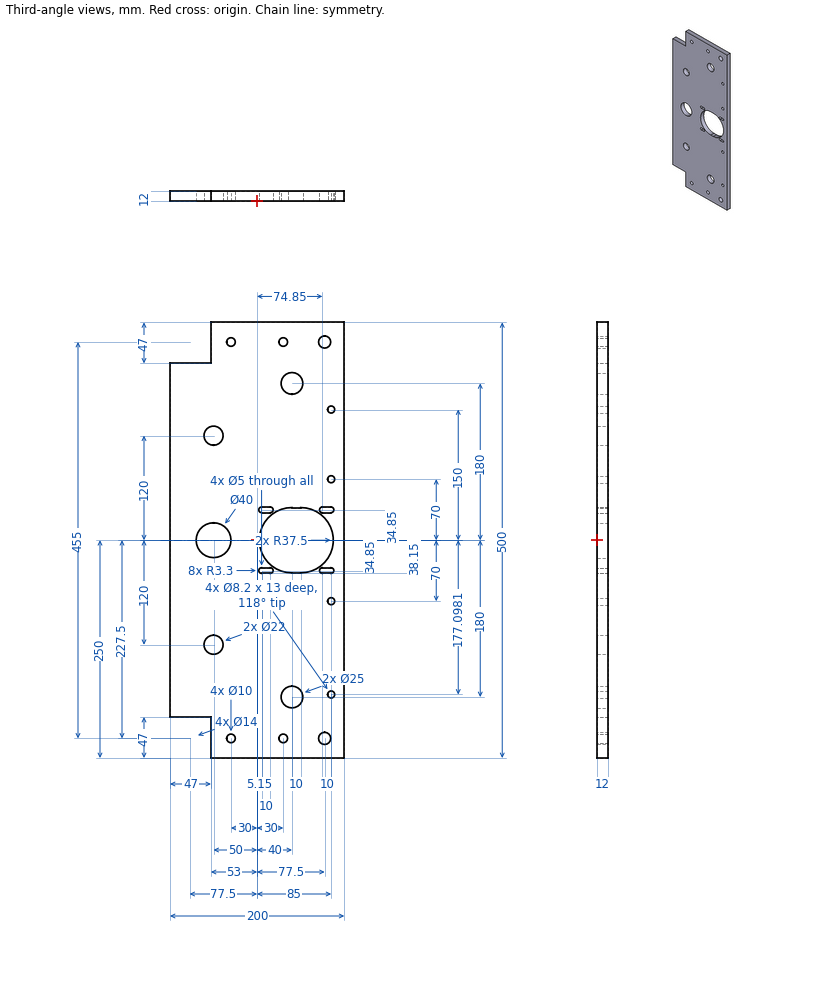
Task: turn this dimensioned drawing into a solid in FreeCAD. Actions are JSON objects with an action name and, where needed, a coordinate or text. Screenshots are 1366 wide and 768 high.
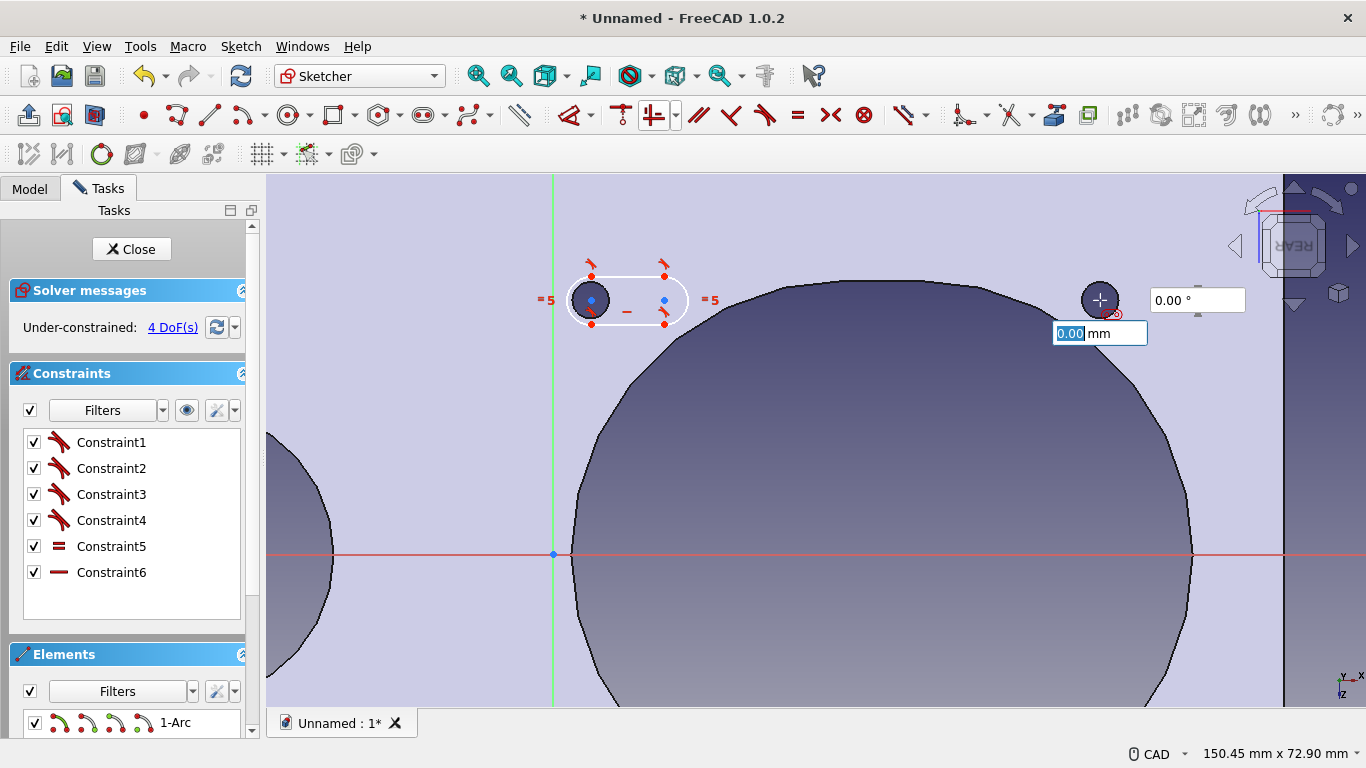
{"action": "left_click", "coordinate": [1173, 300]}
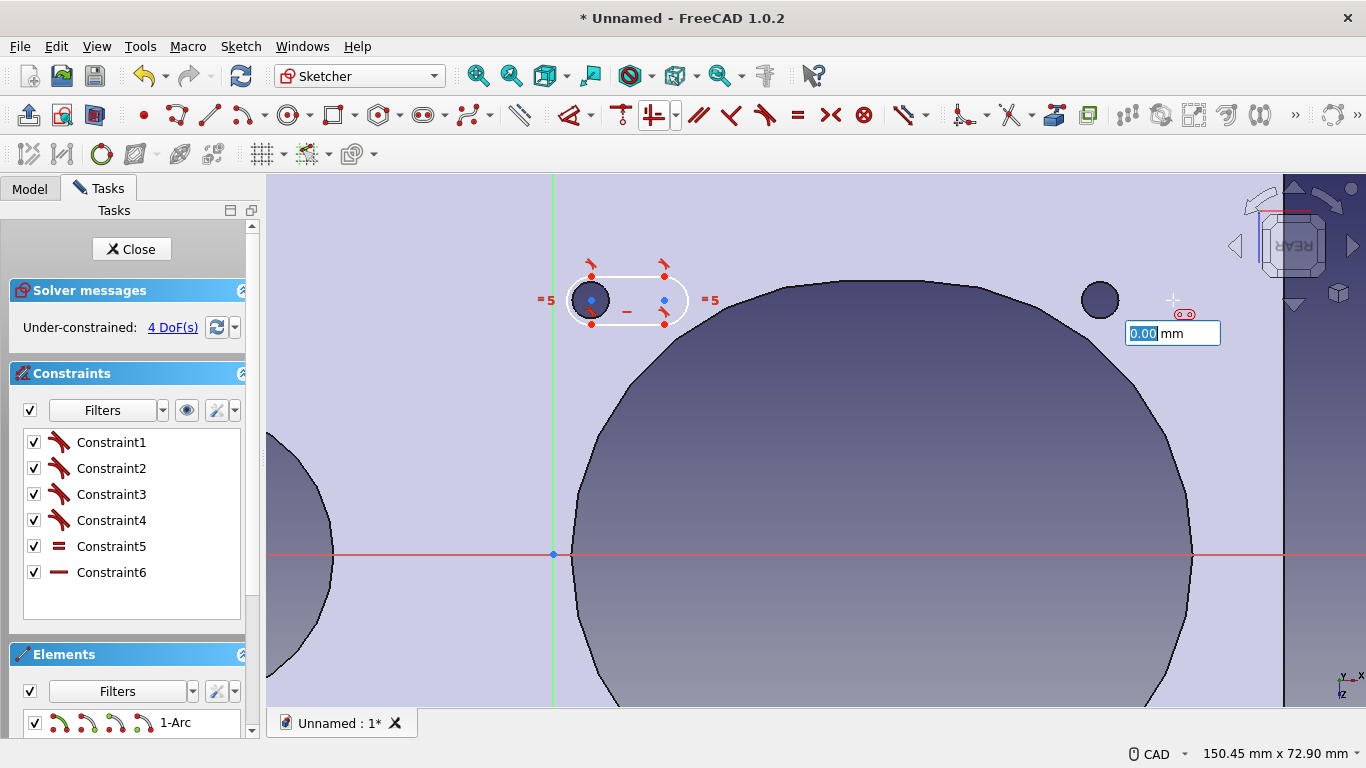
{"action": "left_click", "coordinate": [1137, 276]}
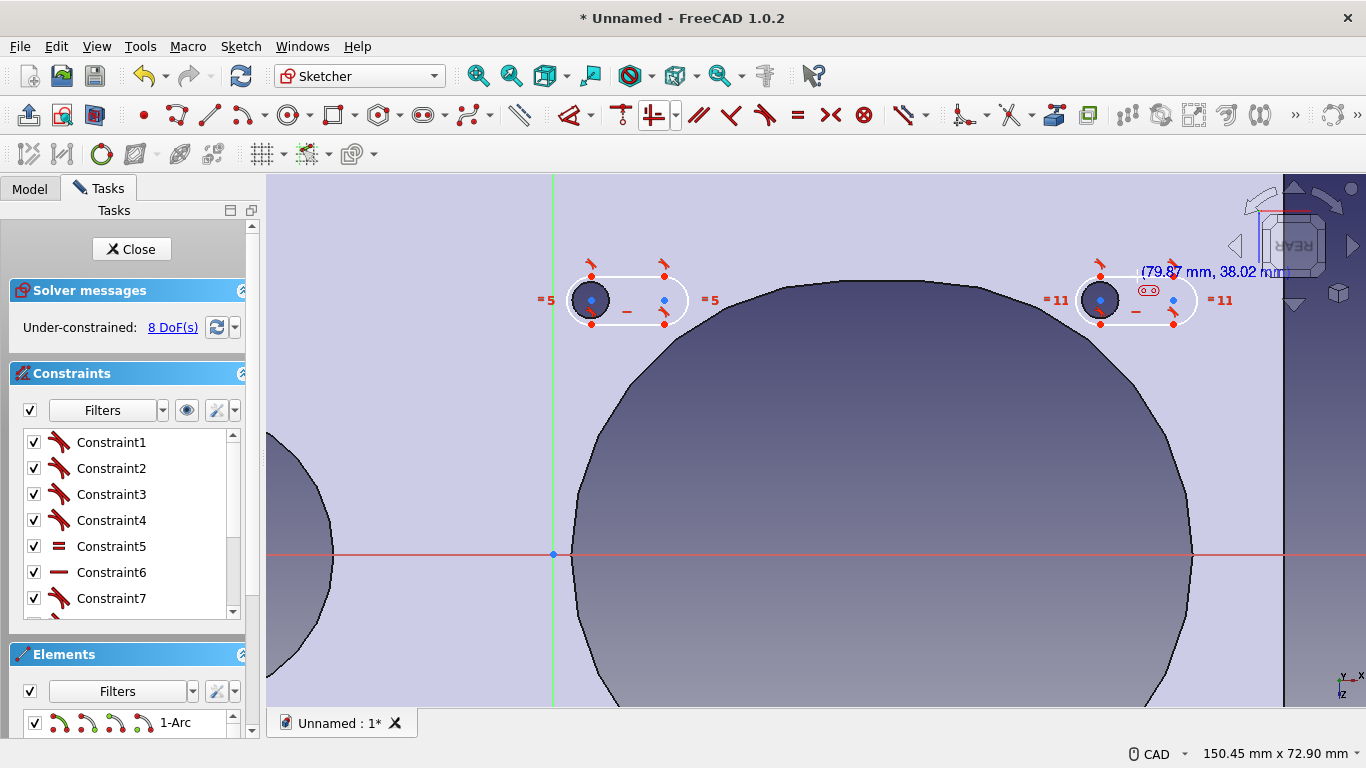
{"action": "scroll", "coordinate": [592, 301], "scroll_direction": "down", "scroll_amount": 3}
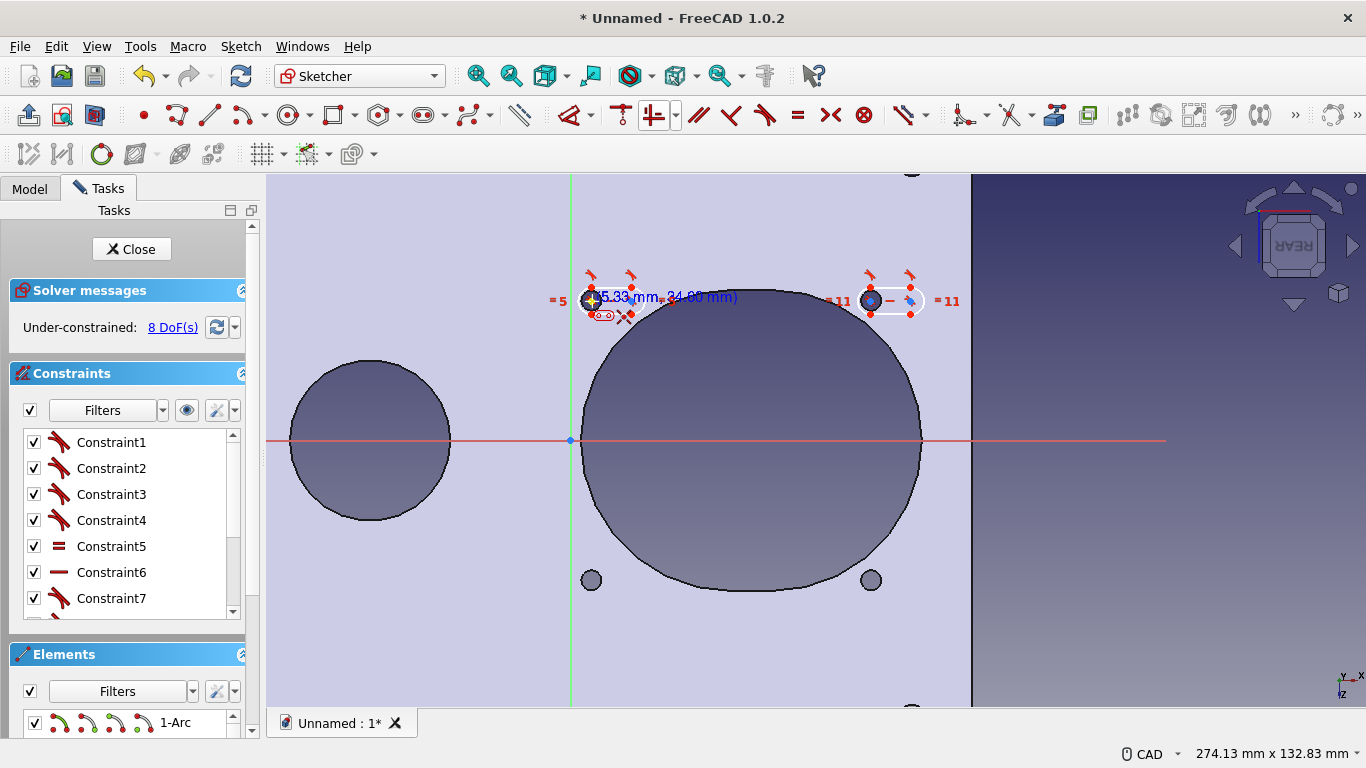
{"action": "scroll", "coordinate": [591, 580], "scroll_direction": "up", "scroll_amount": 3}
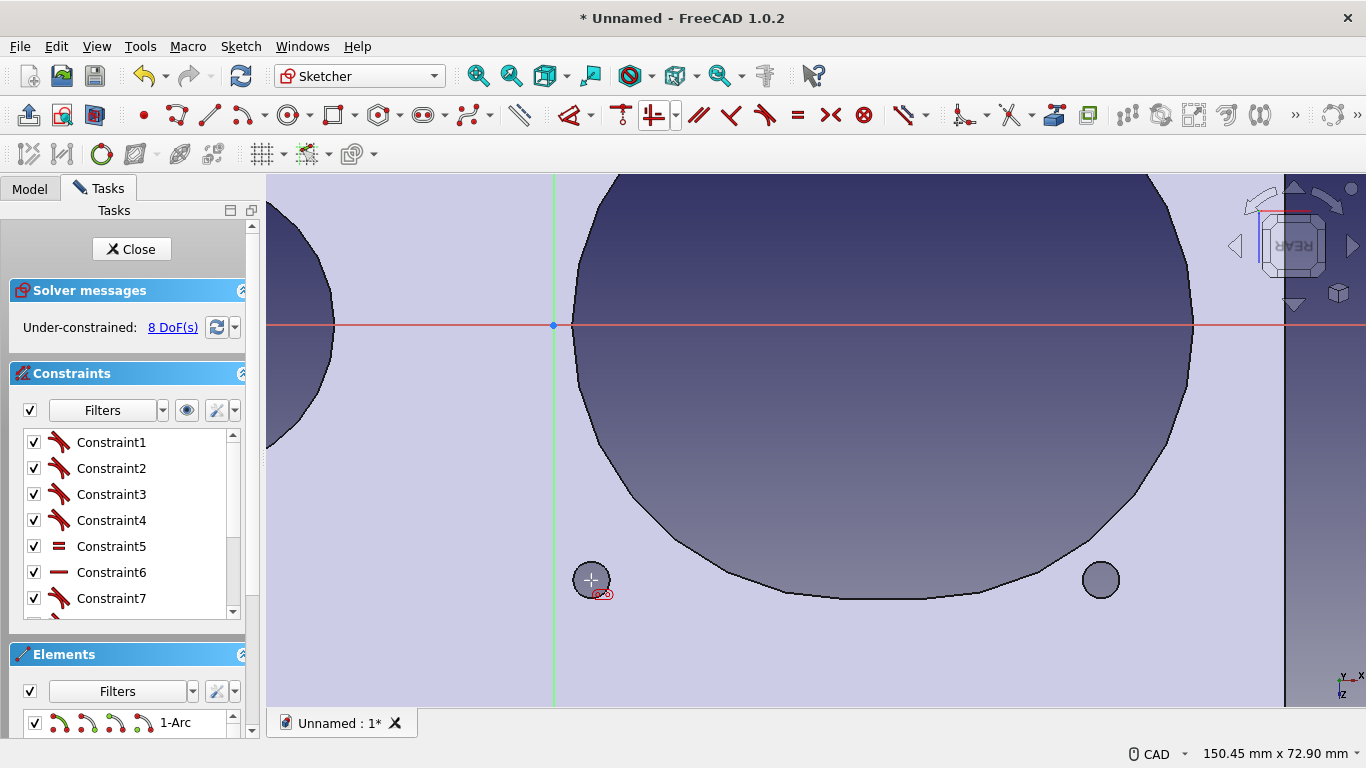
{"action": "left_click", "coordinate": [591, 580]}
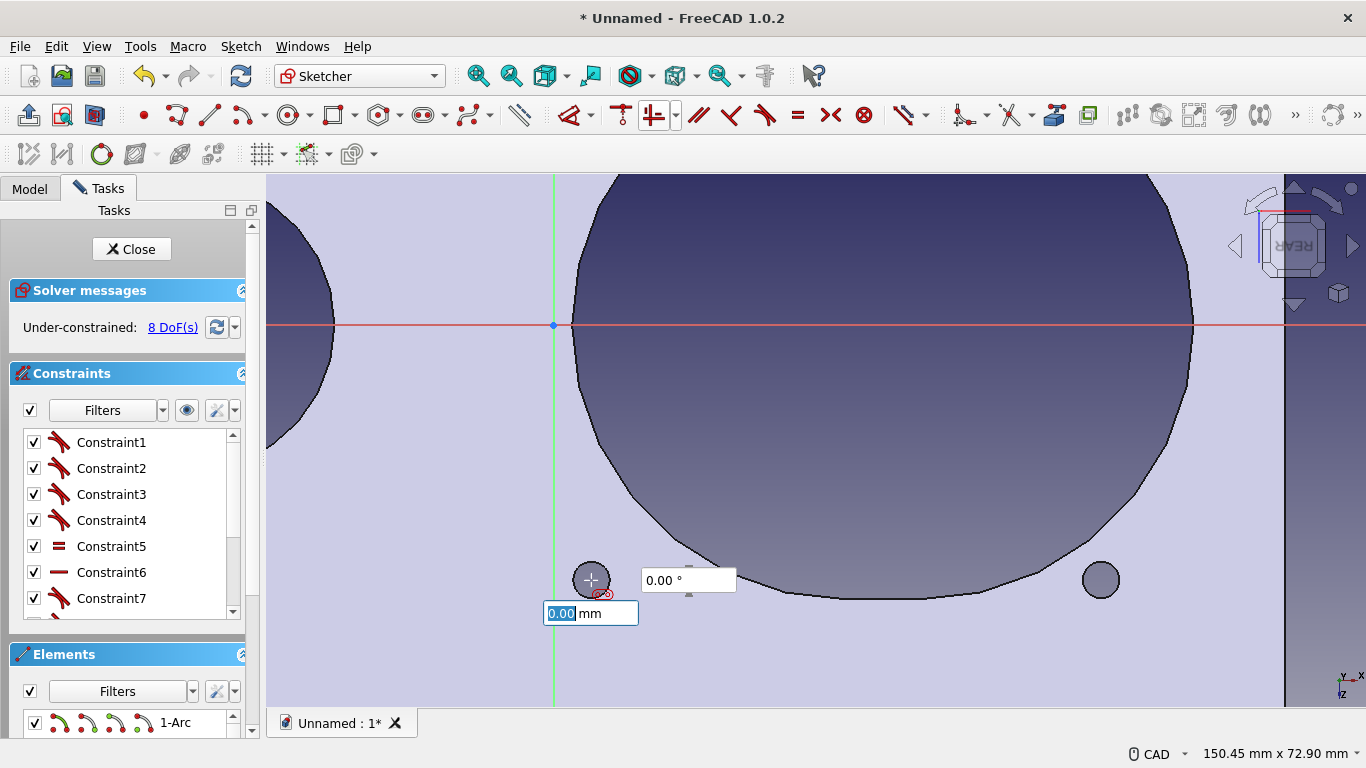
{"action": "left_click", "coordinate": [665, 580]}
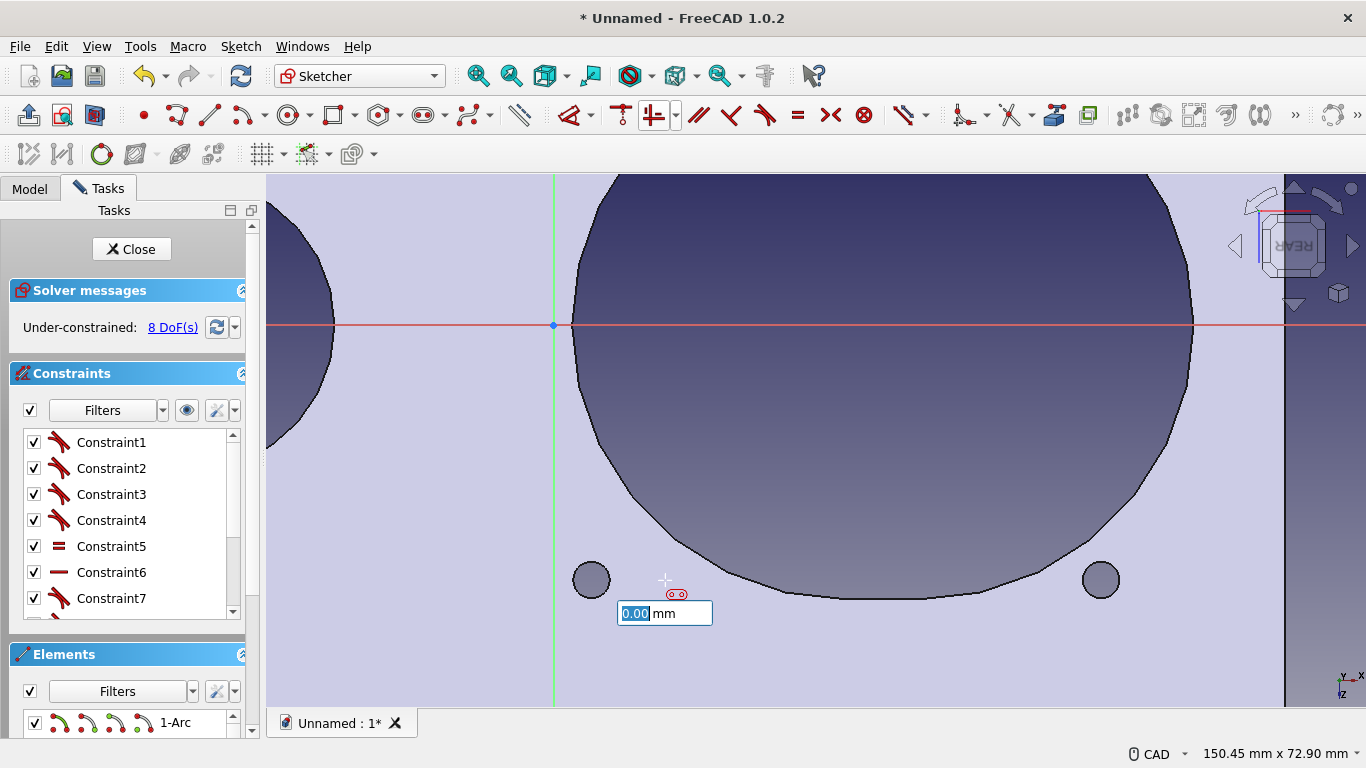
{"action": "left_click", "coordinate": [628, 556]}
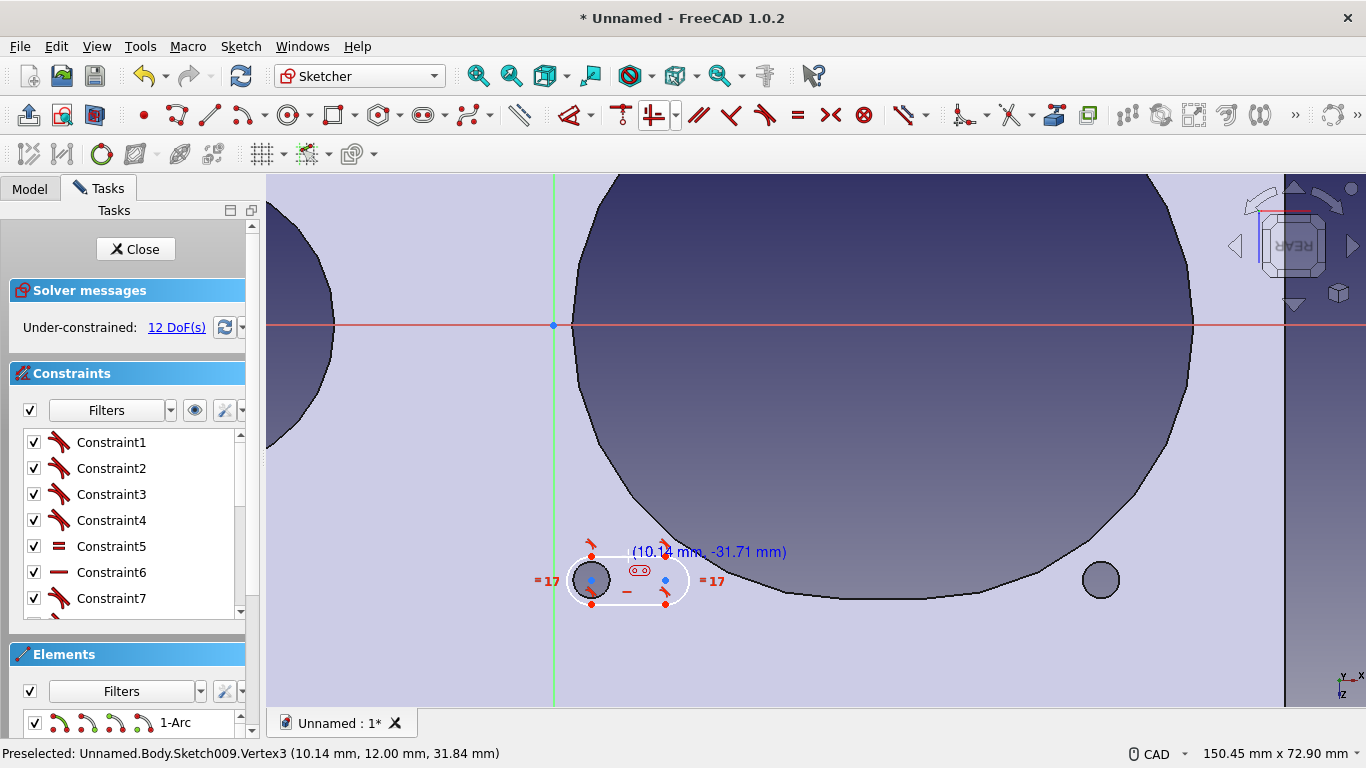
{"action": "left_click", "coordinate": [1101, 580]}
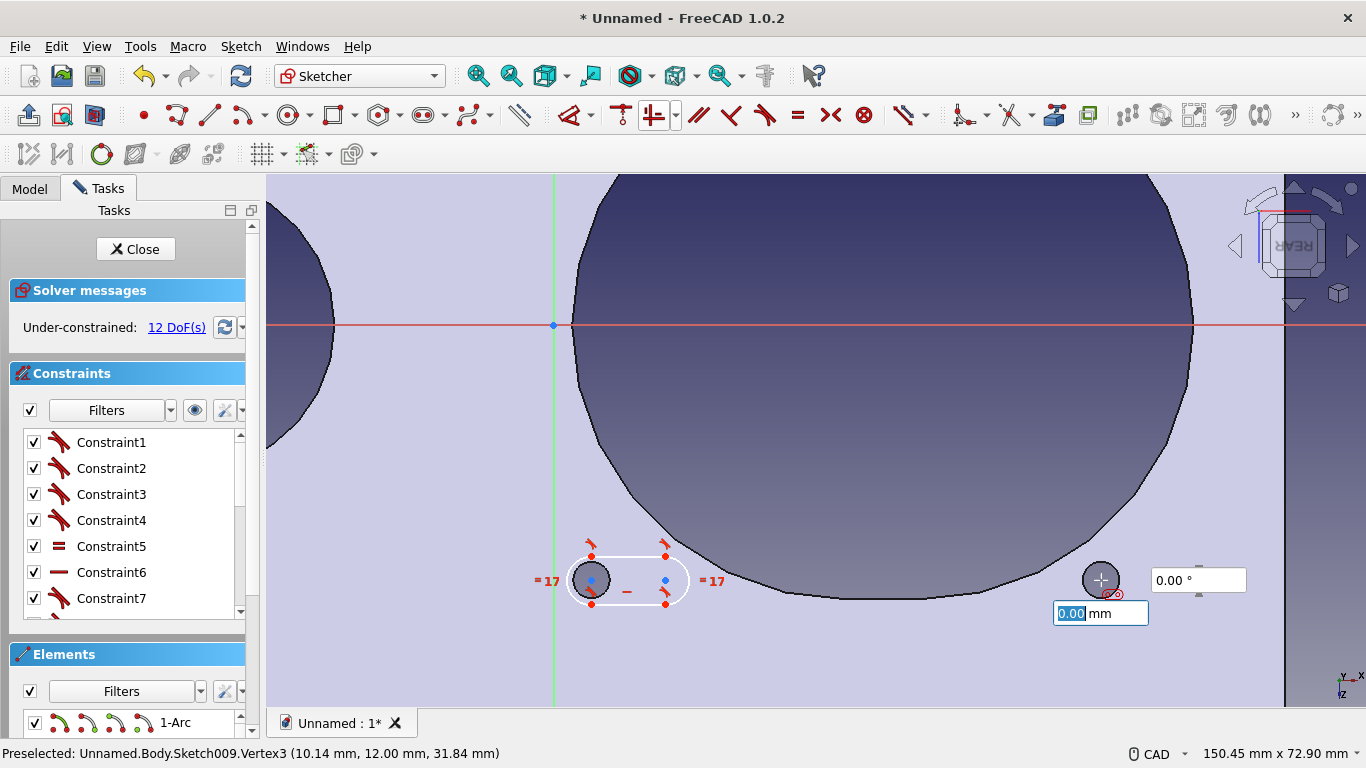
{"action": "left_click", "coordinate": [1174, 580]}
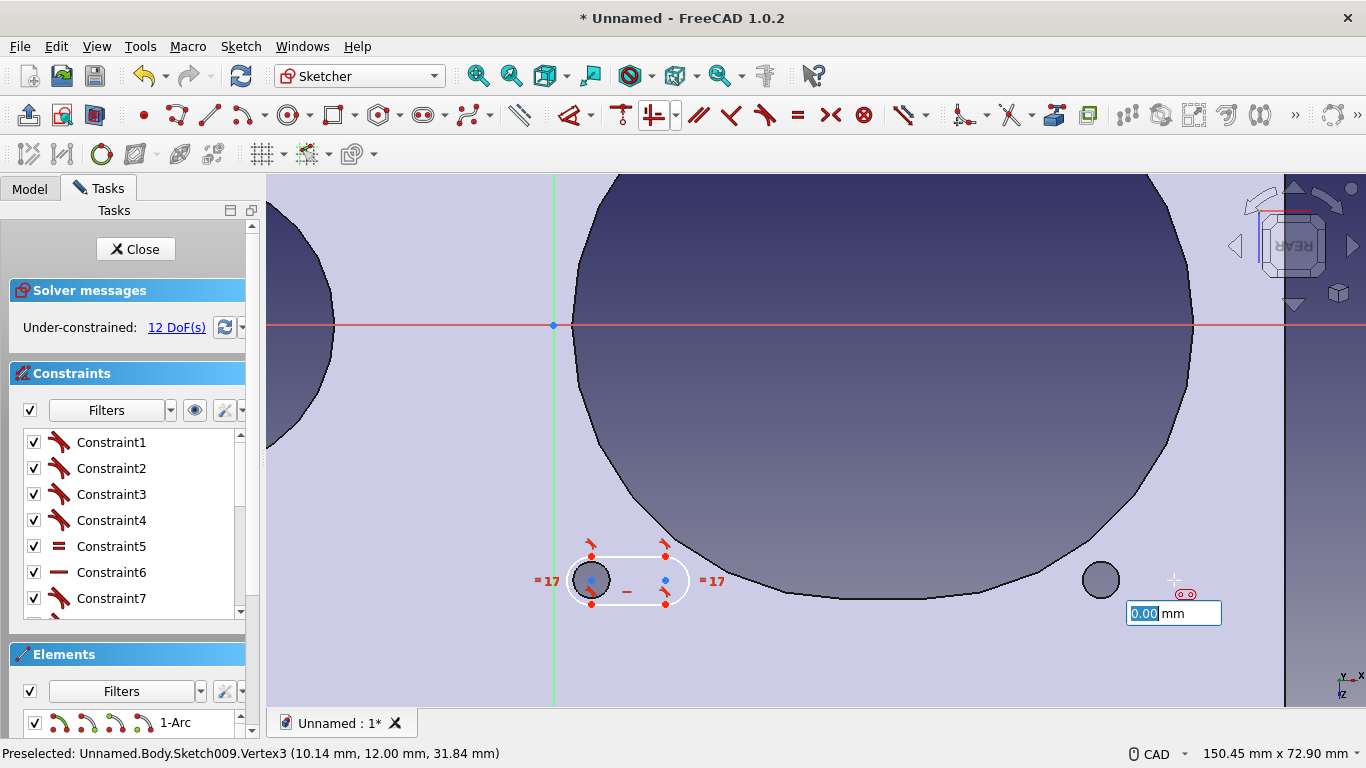
{"action": "left_click", "coordinate": [1138, 556]}
{"action": "key", "text": "Escape"}